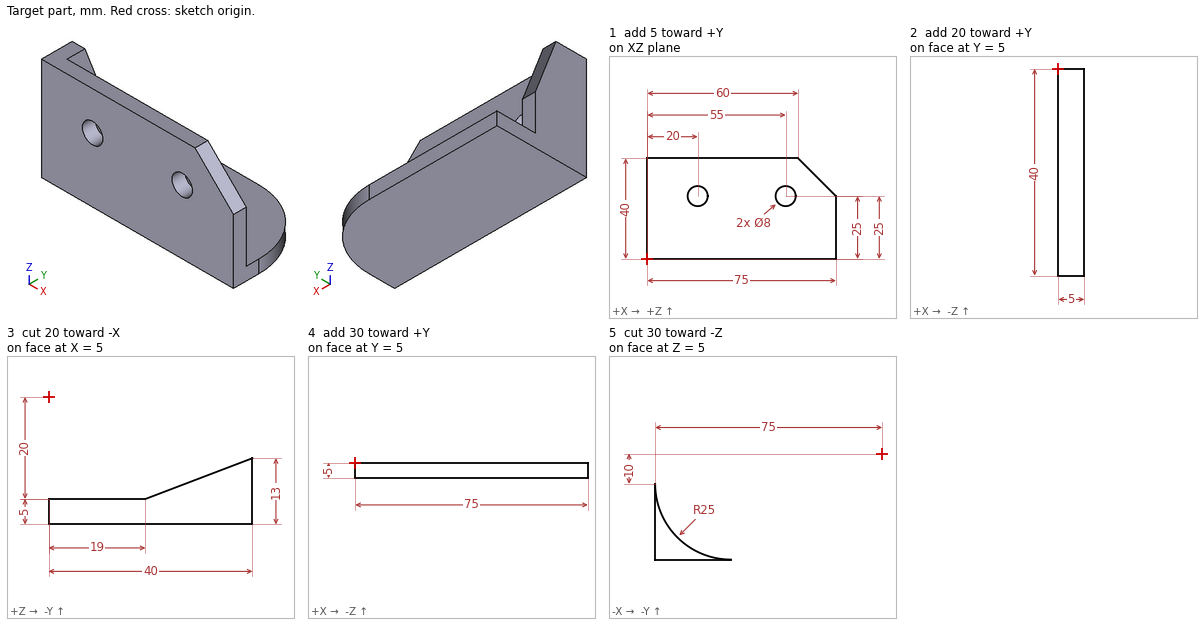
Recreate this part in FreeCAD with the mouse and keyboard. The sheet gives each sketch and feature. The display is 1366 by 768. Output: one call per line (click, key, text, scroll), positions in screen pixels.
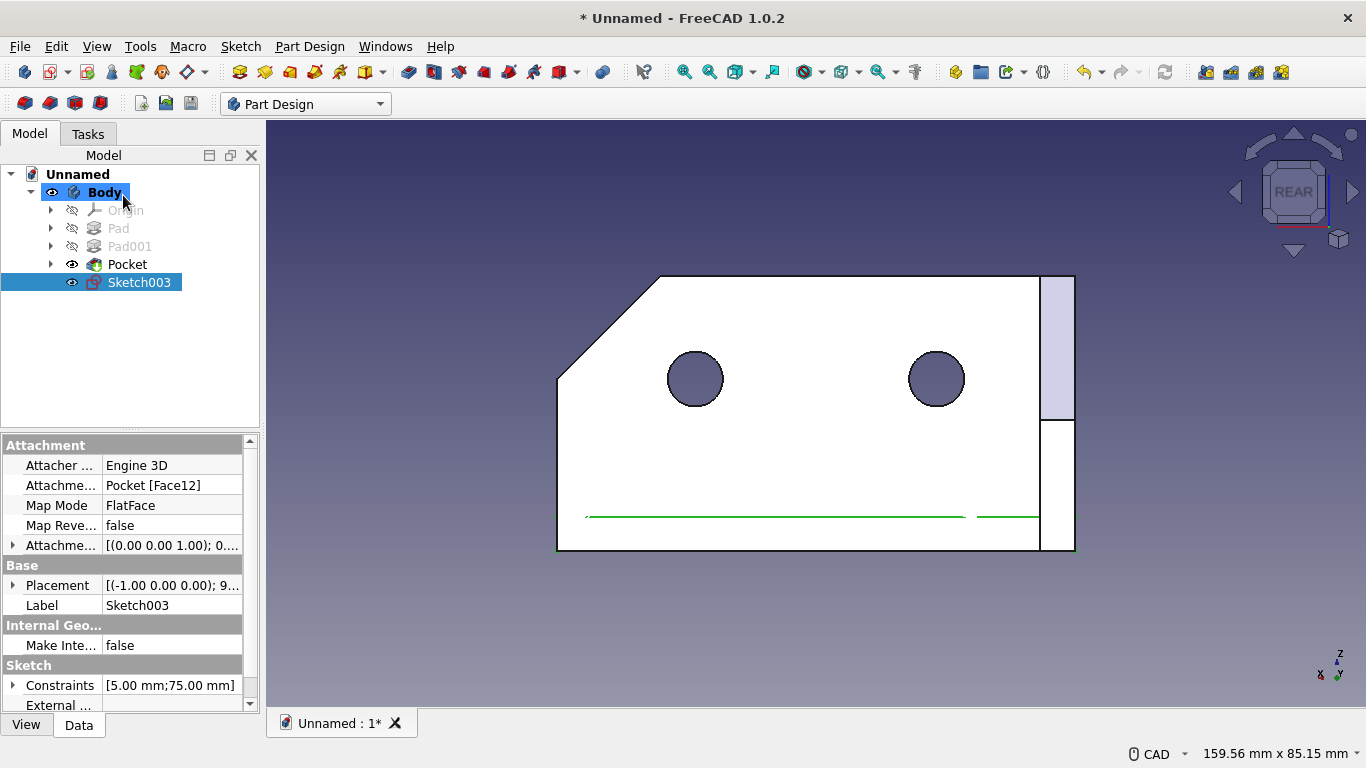
click(240, 72)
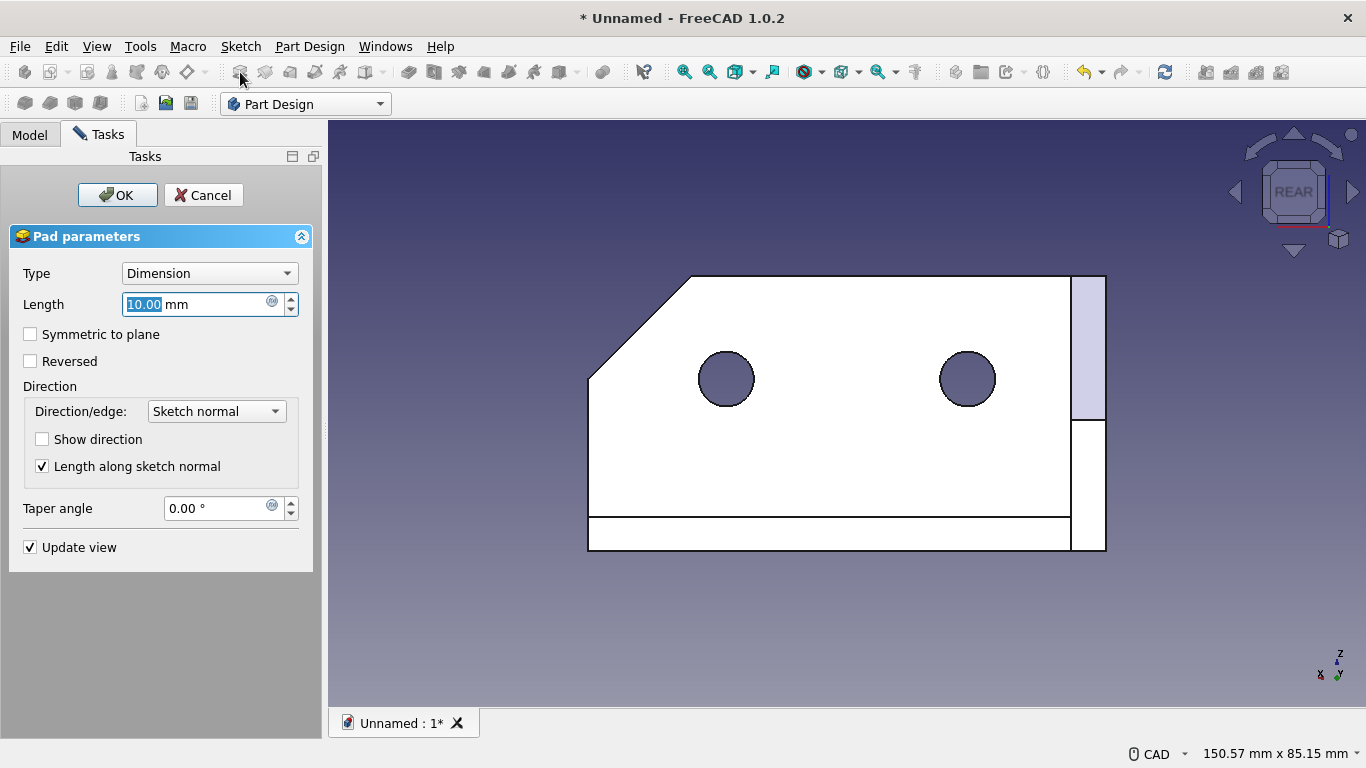
text(30)
key(Tab)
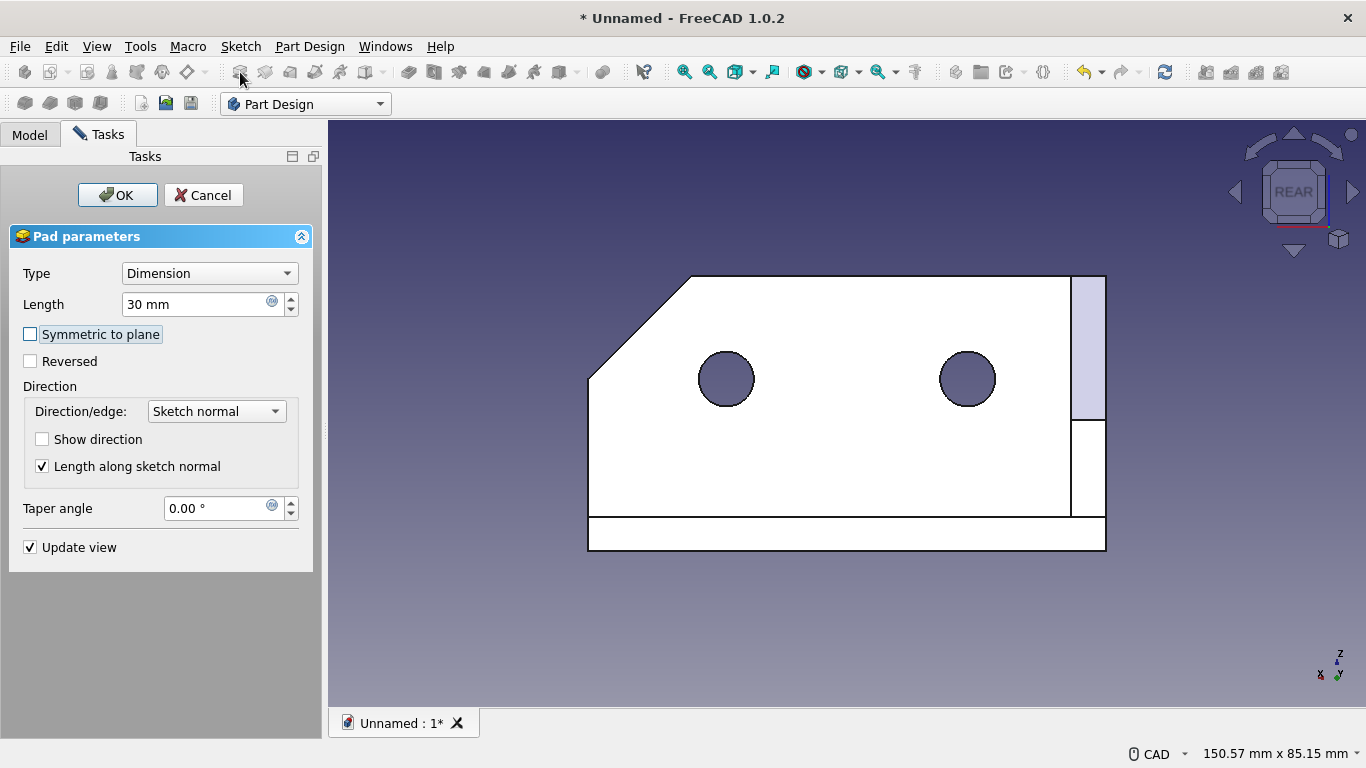
click(118, 195)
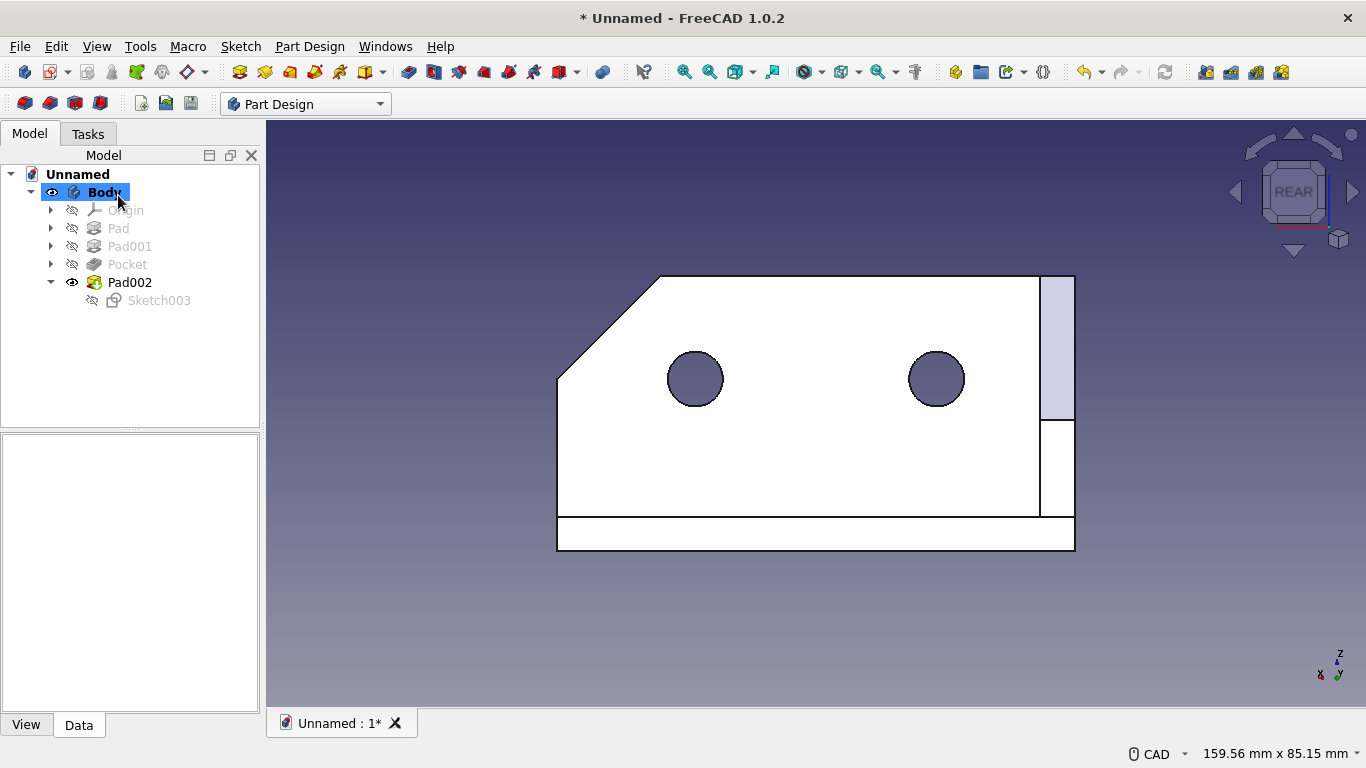
key(0)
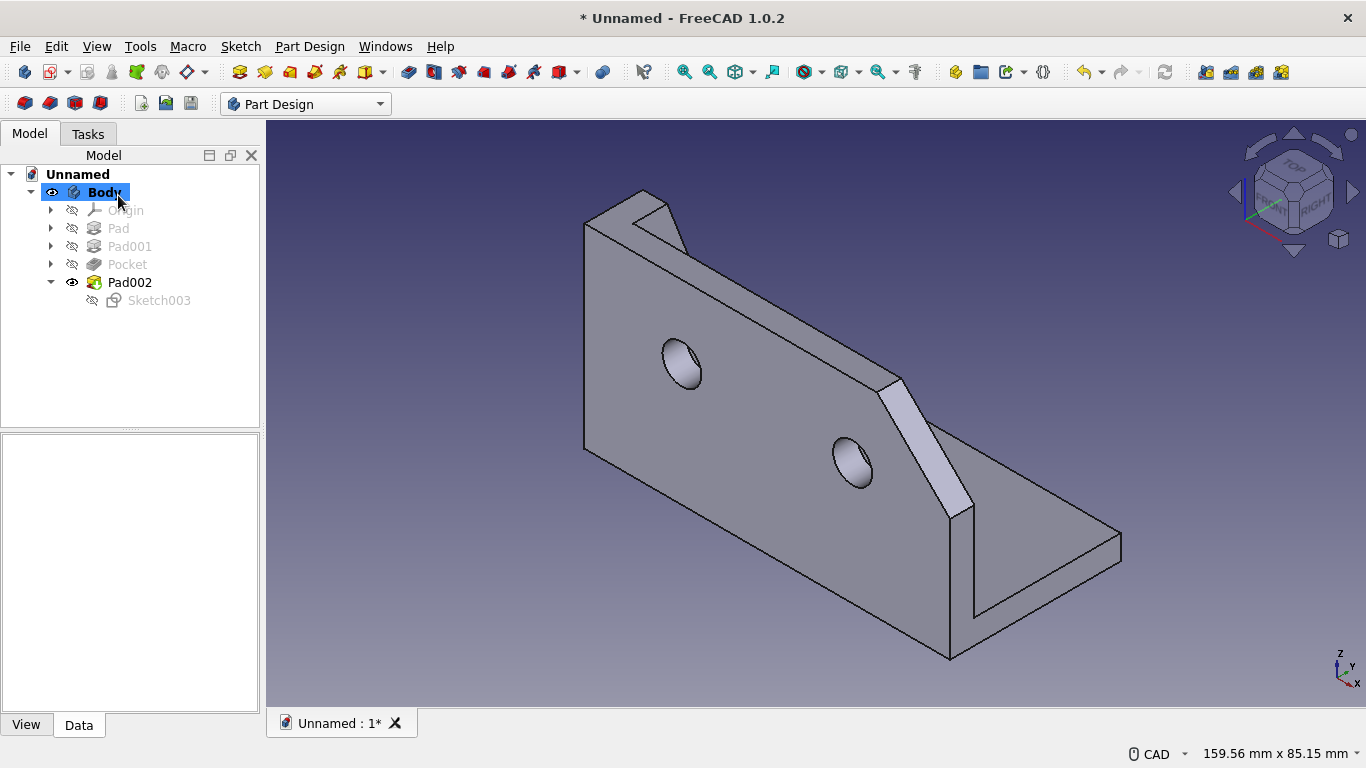
click(990, 517)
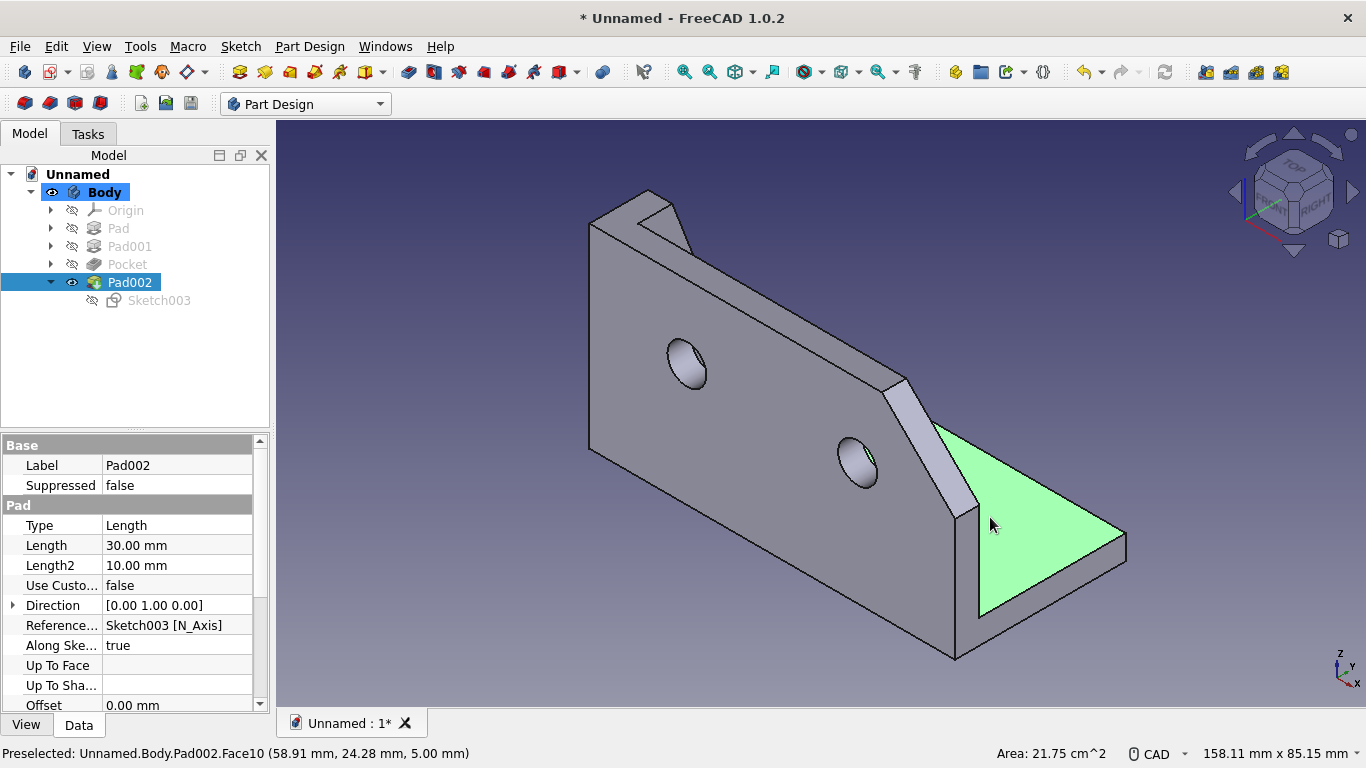
click(50, 72)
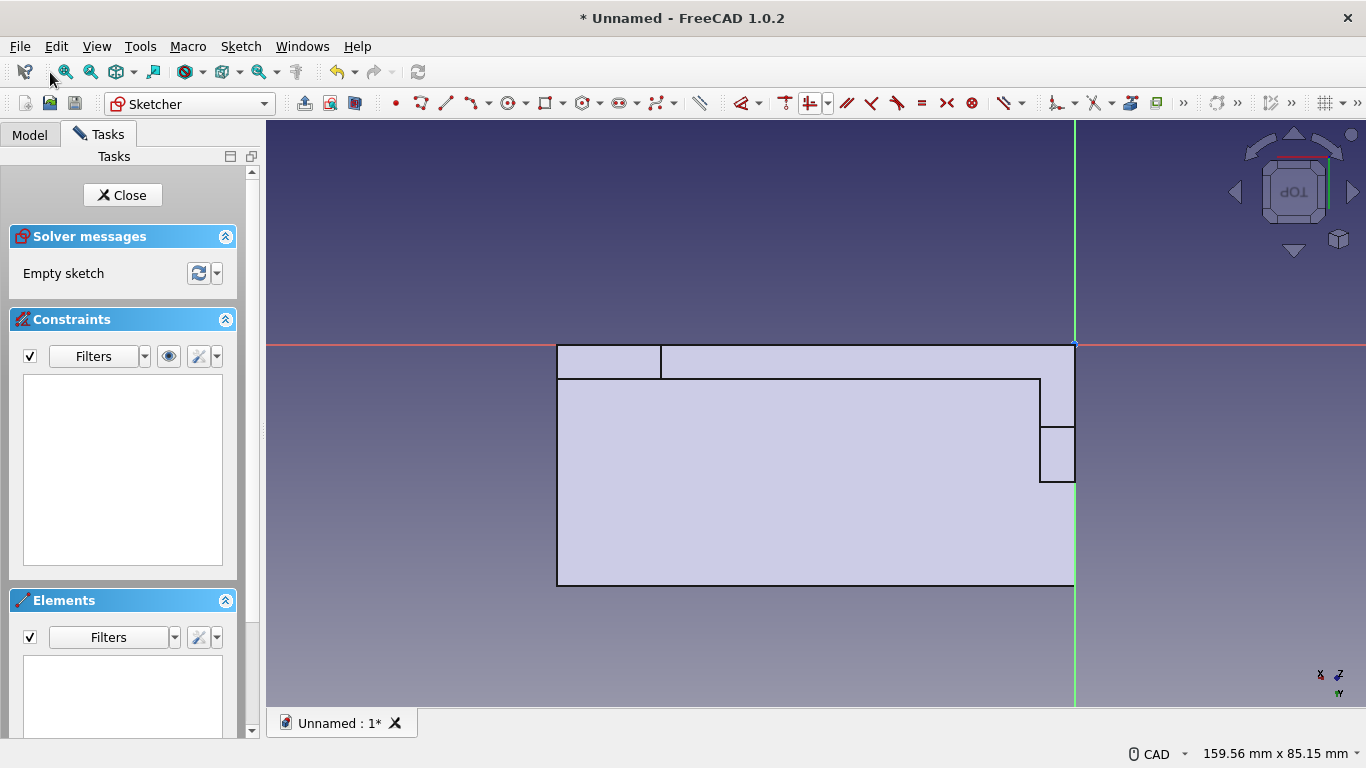
click(355, 104)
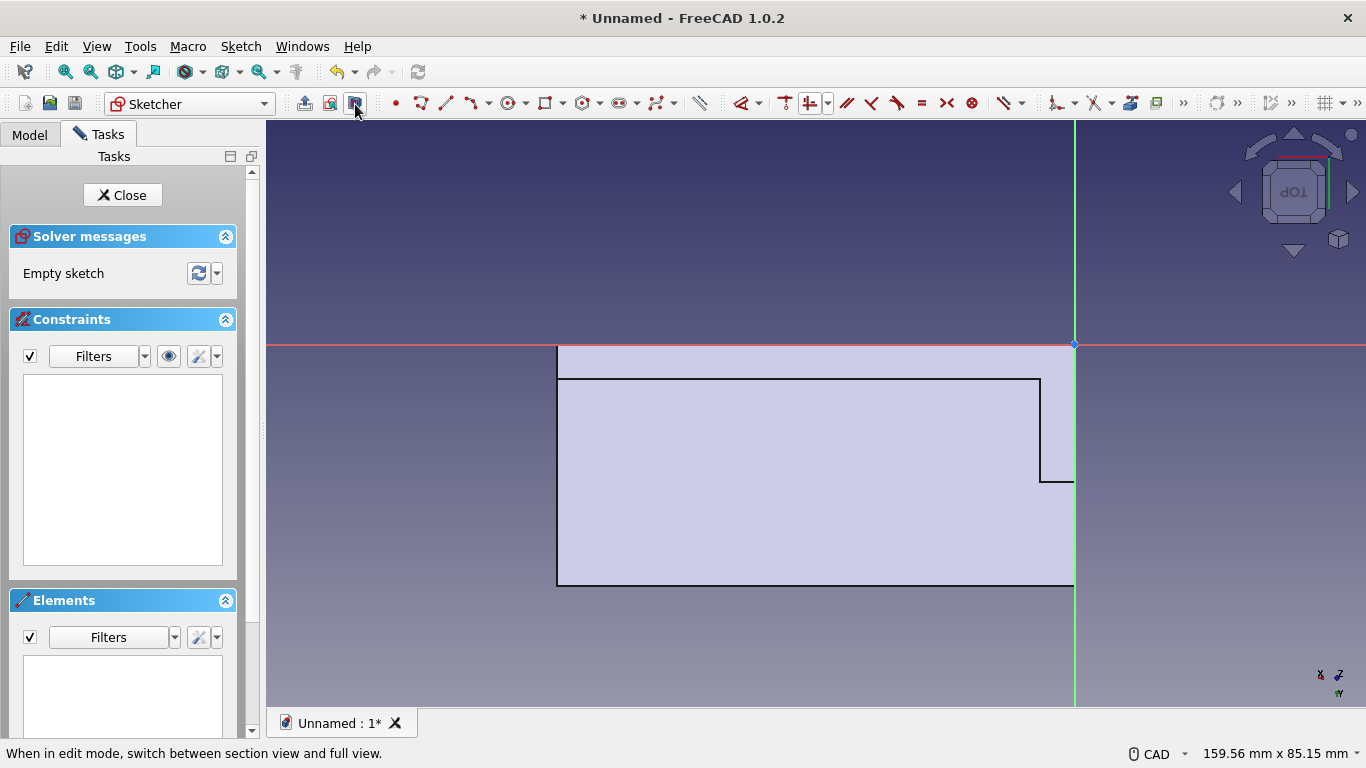
scroll(559, 570, up, 4)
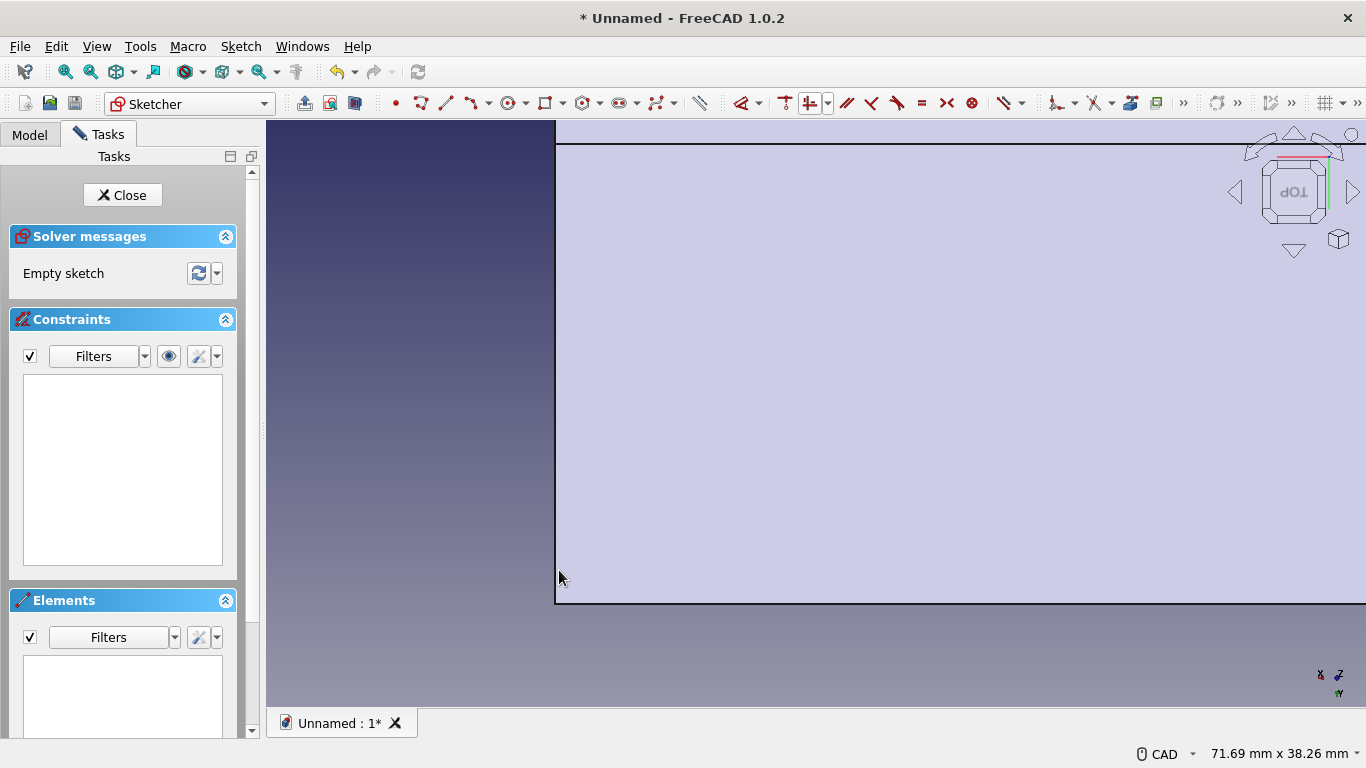
click(421, 104)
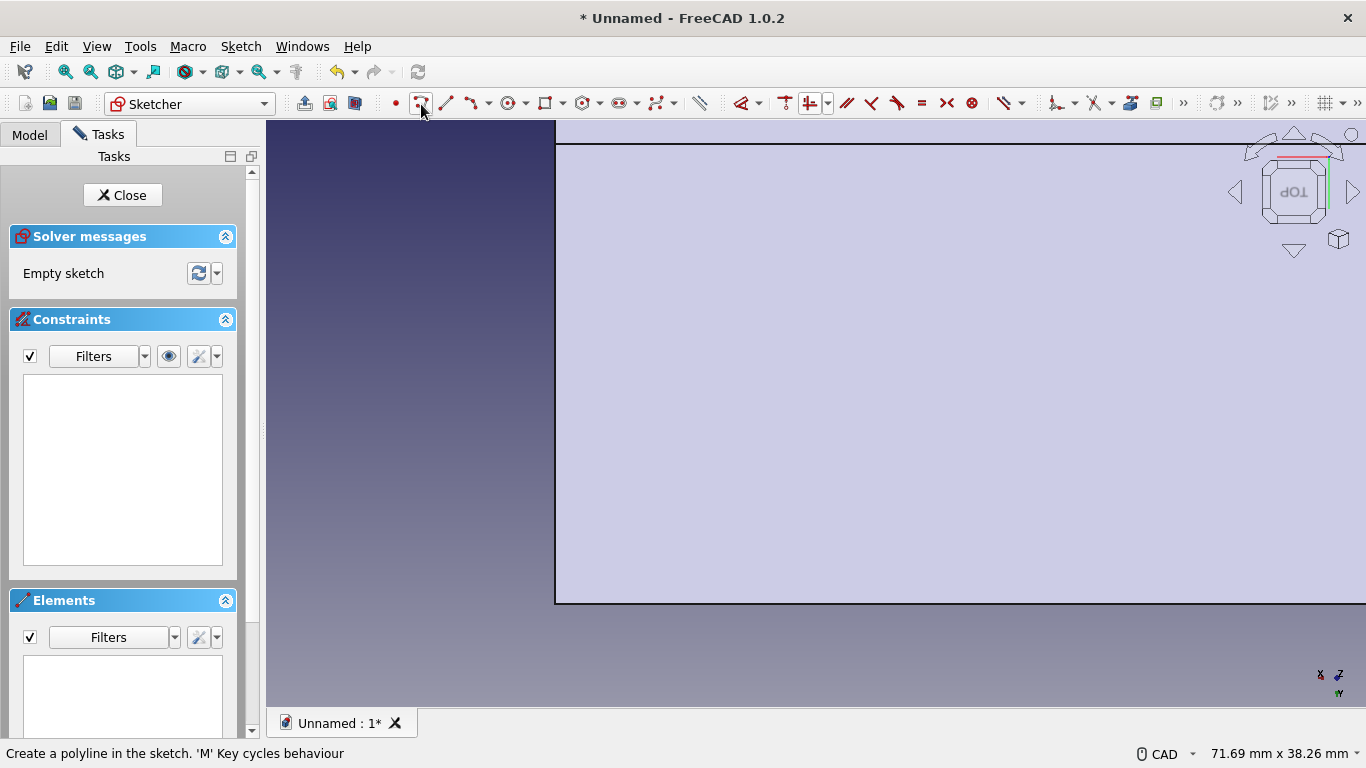
click(555, 221)
click(555, 604)
click(939, 604)
right_click(939, 604)